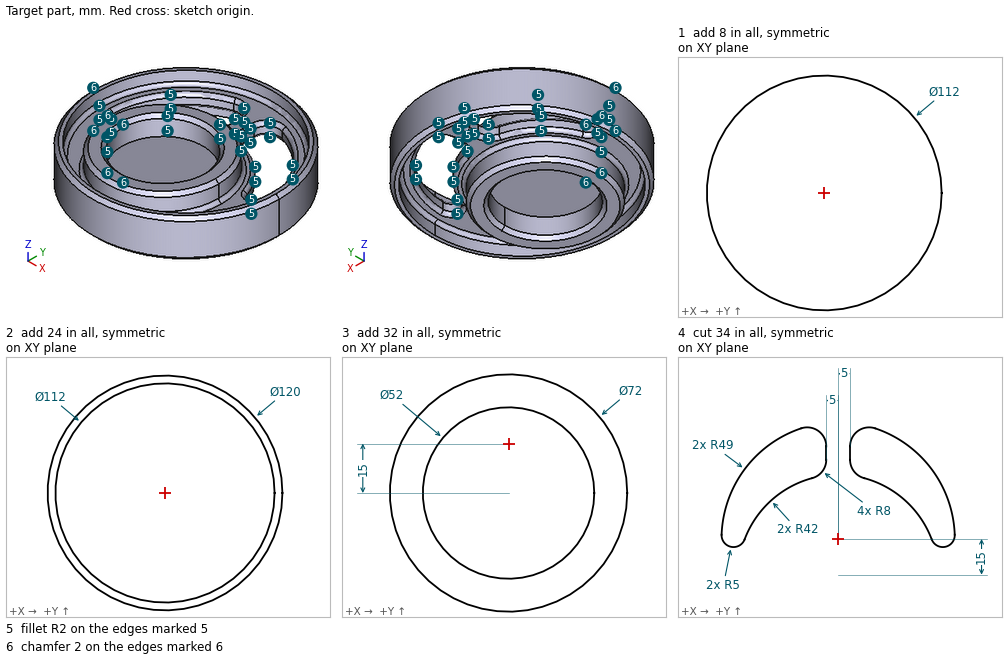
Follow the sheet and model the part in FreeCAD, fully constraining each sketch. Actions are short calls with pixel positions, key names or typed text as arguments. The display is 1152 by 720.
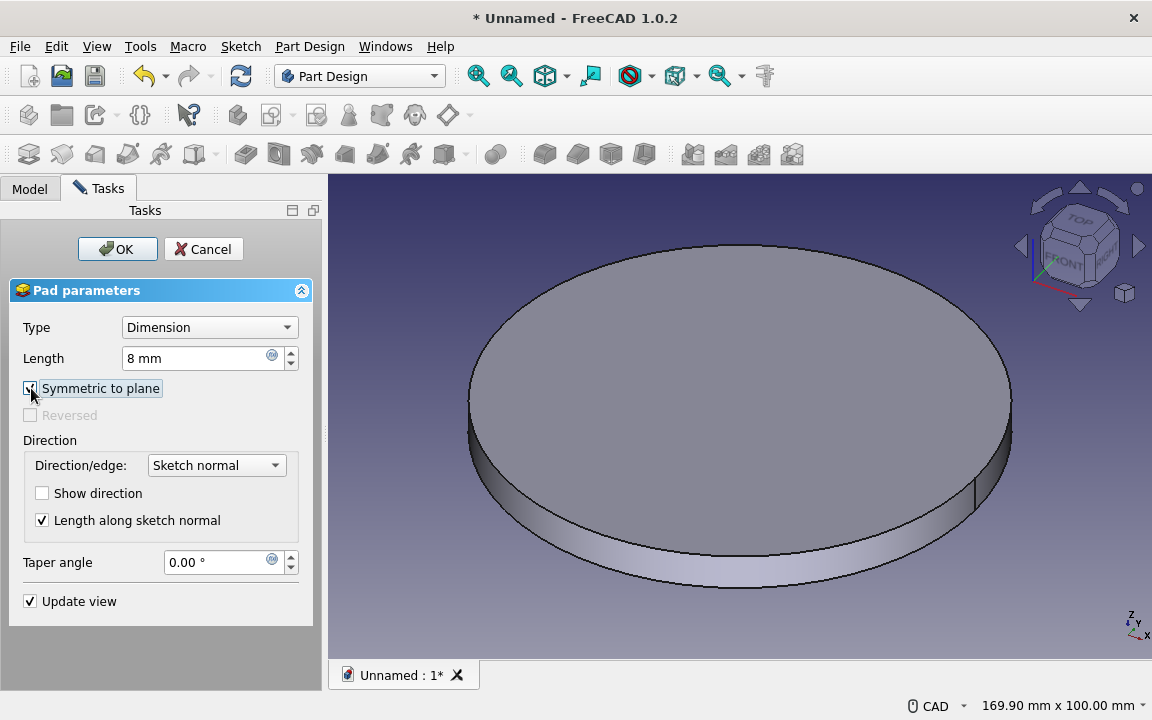
click(118, 249)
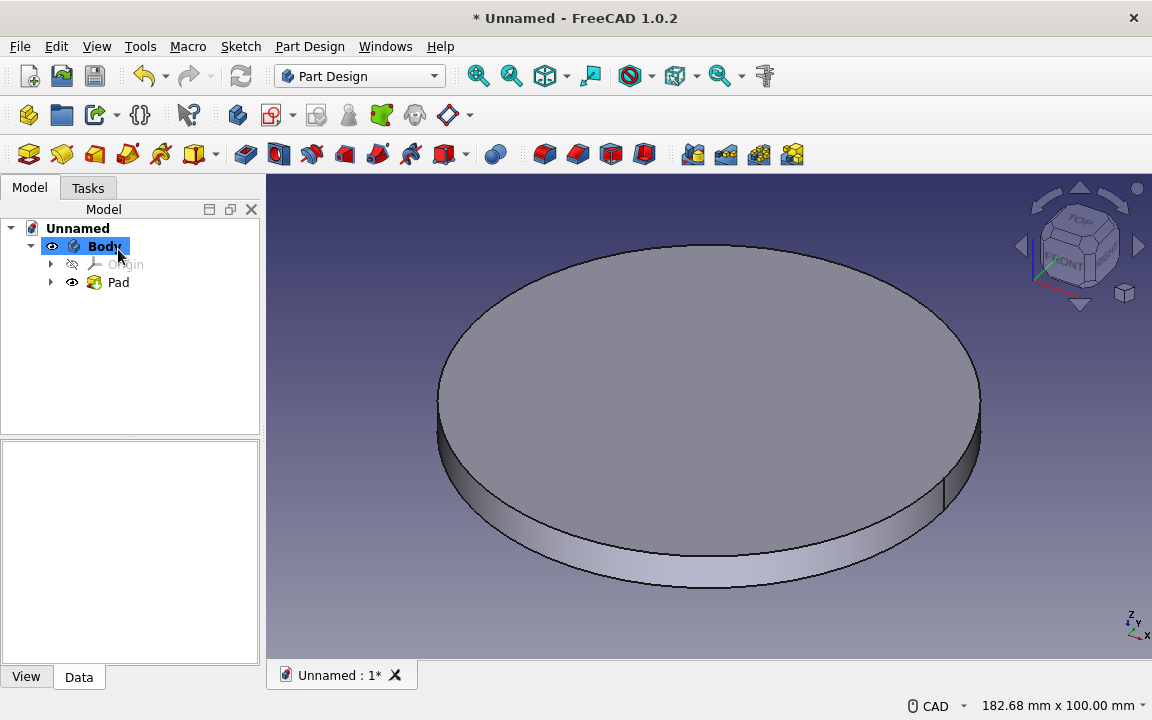
click(270, 116)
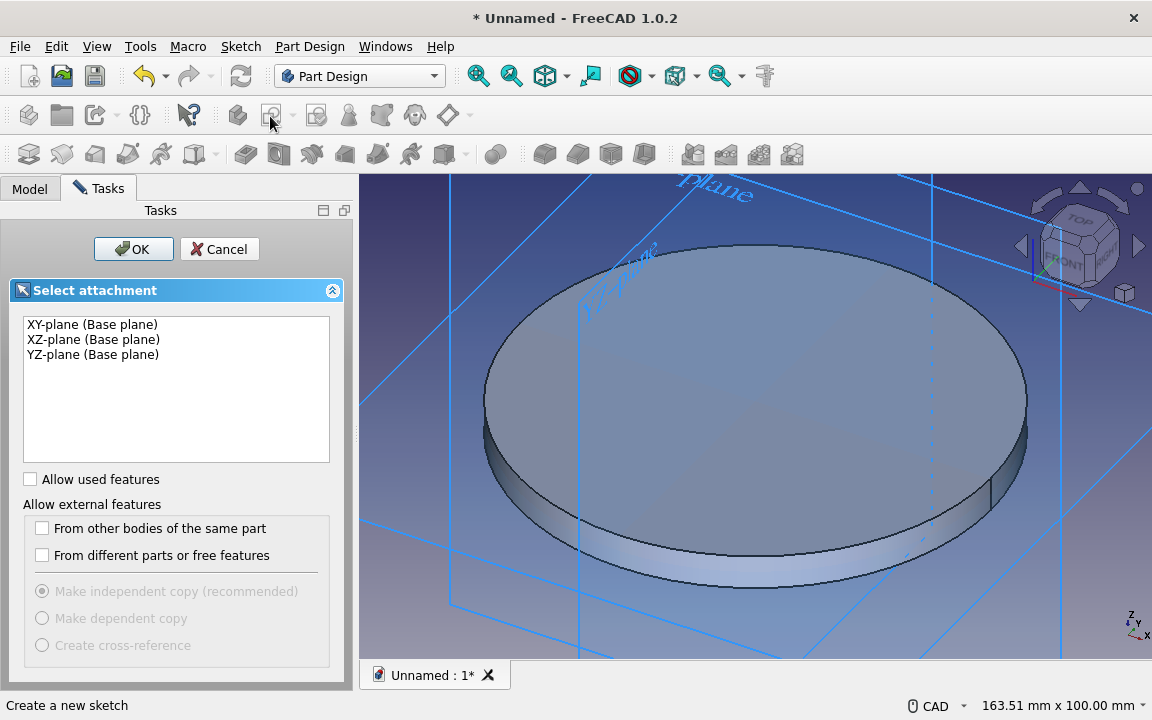
click(84, 324)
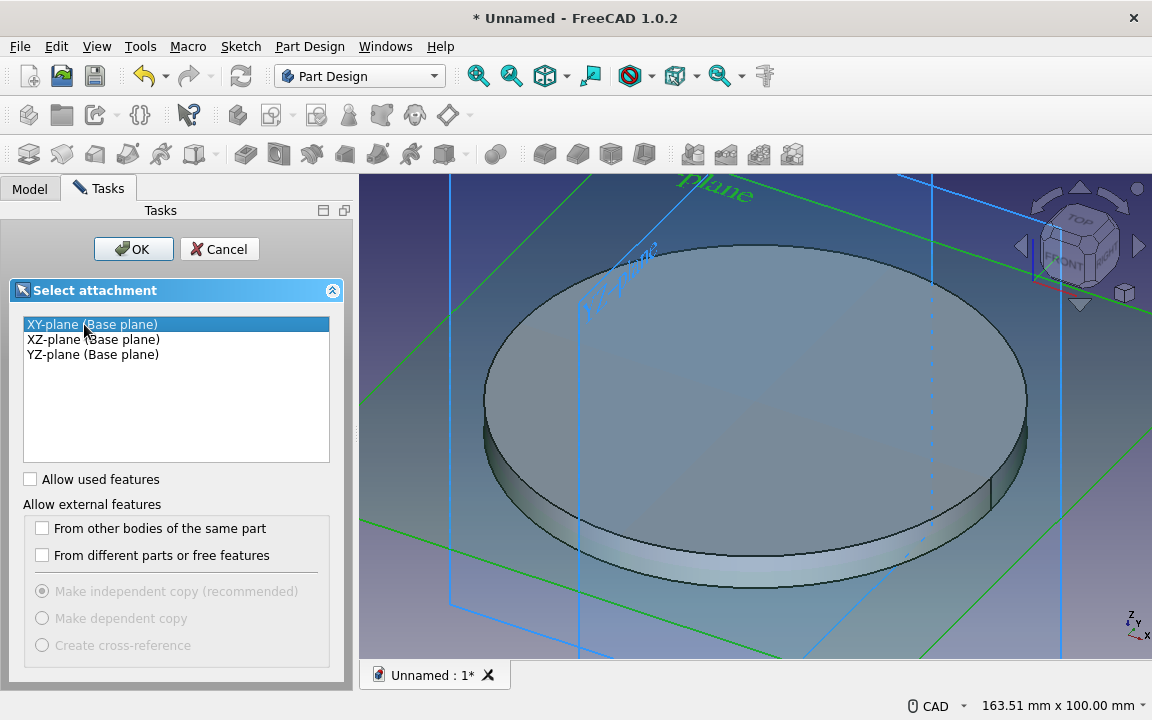
click(134, 249)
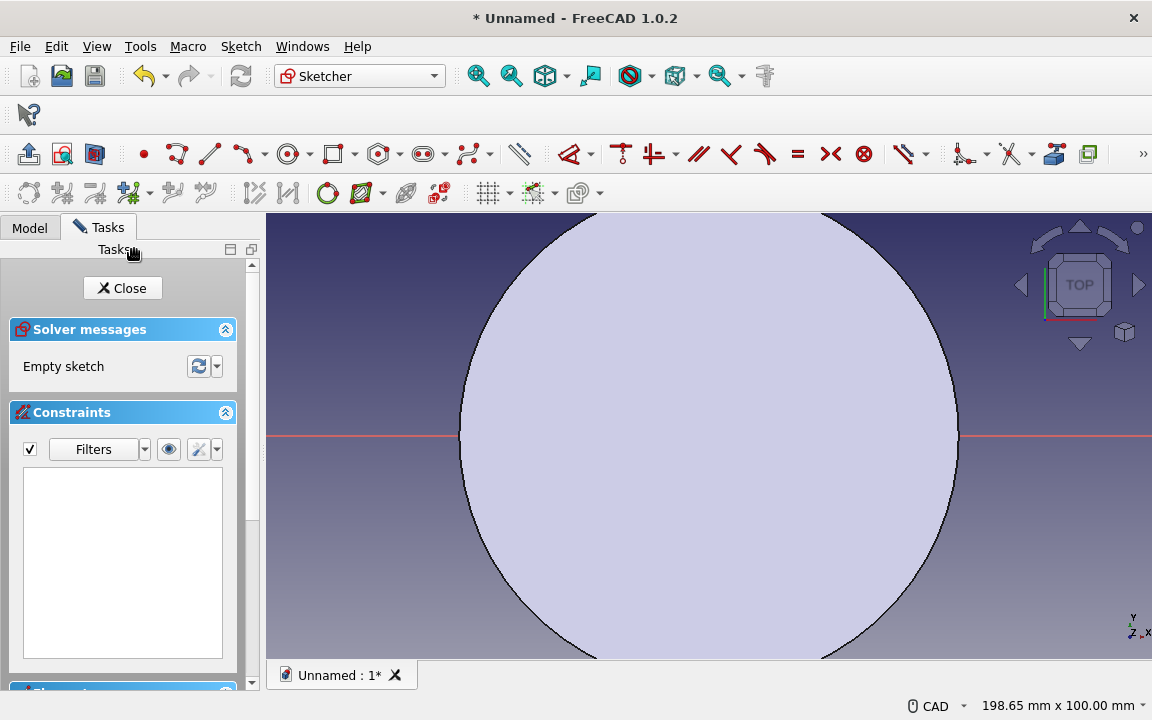
key(q)
key(s)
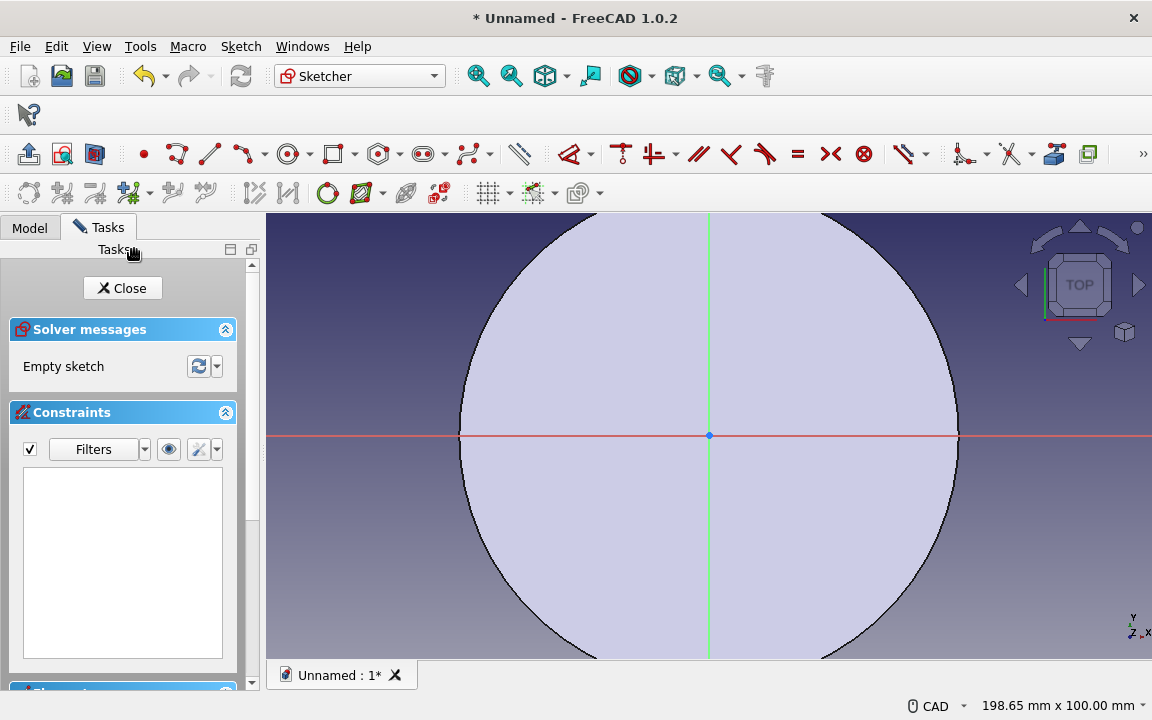
scroll(557, 436, down, 3)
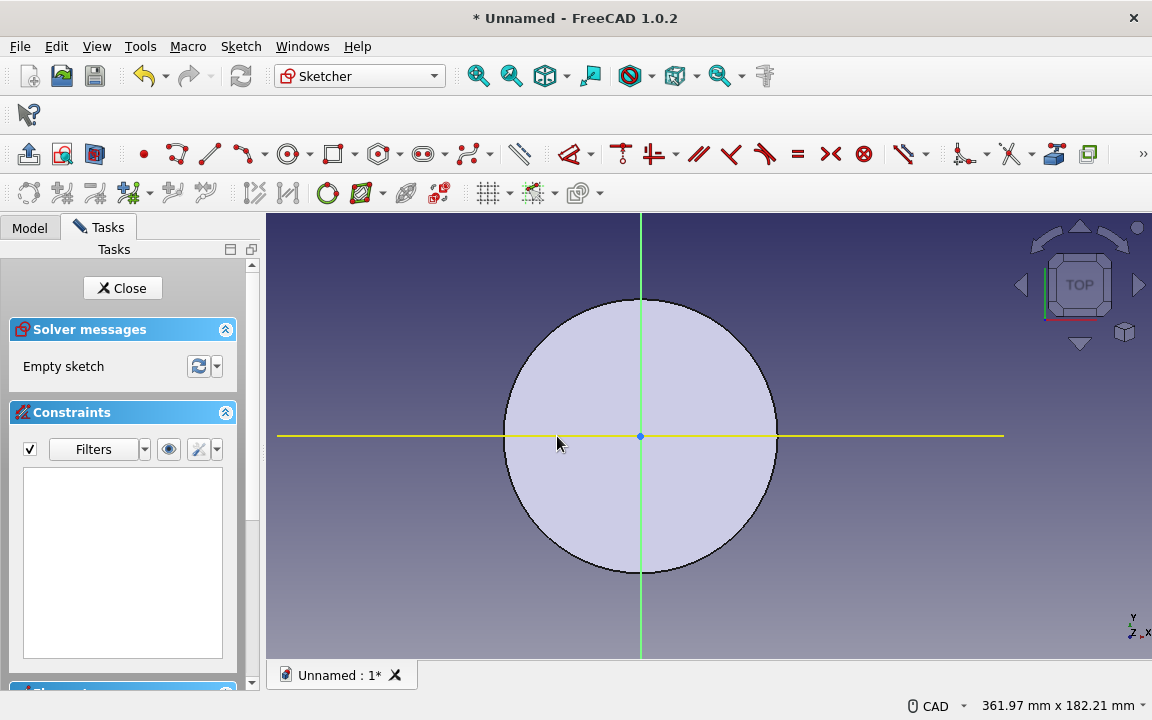
key(g)
key(c)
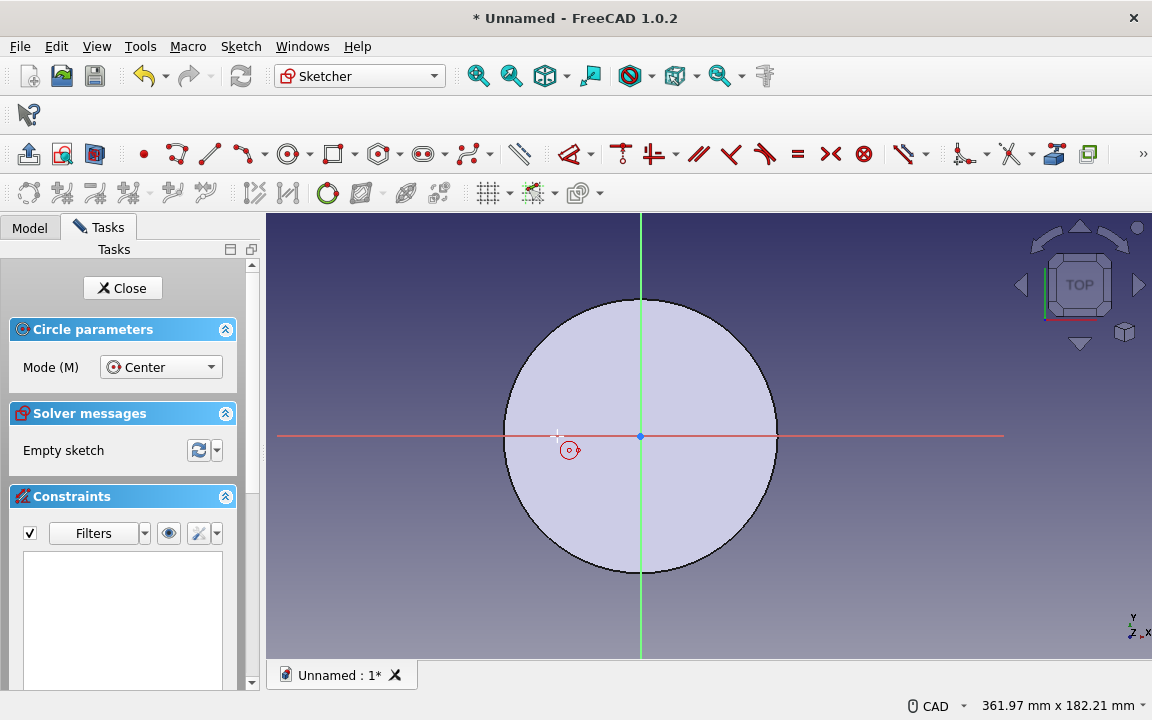
click(641, 436)
move(744, 332)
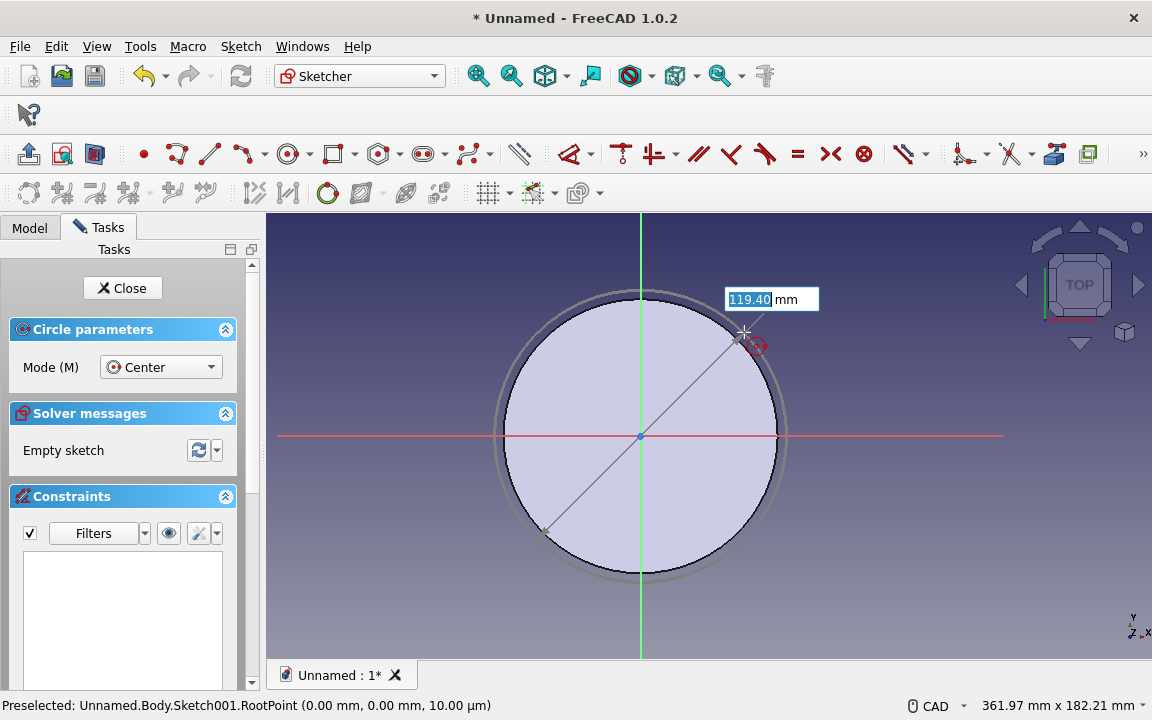
text(120)
key(Return)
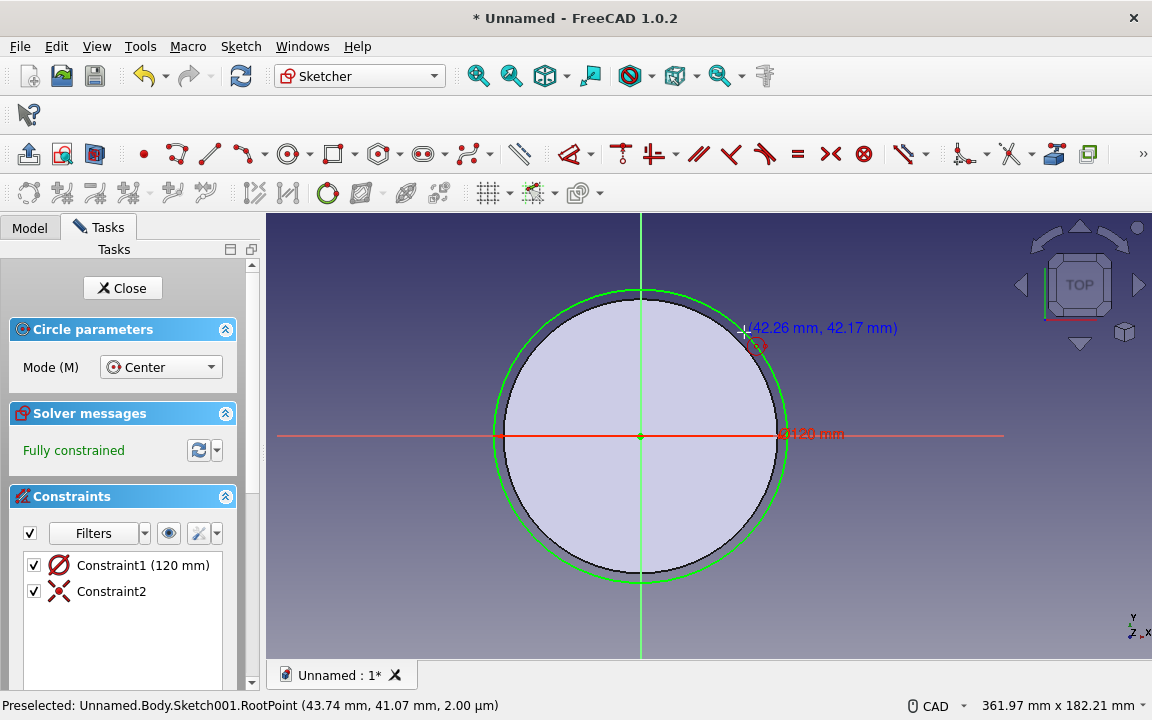
click(641, 436)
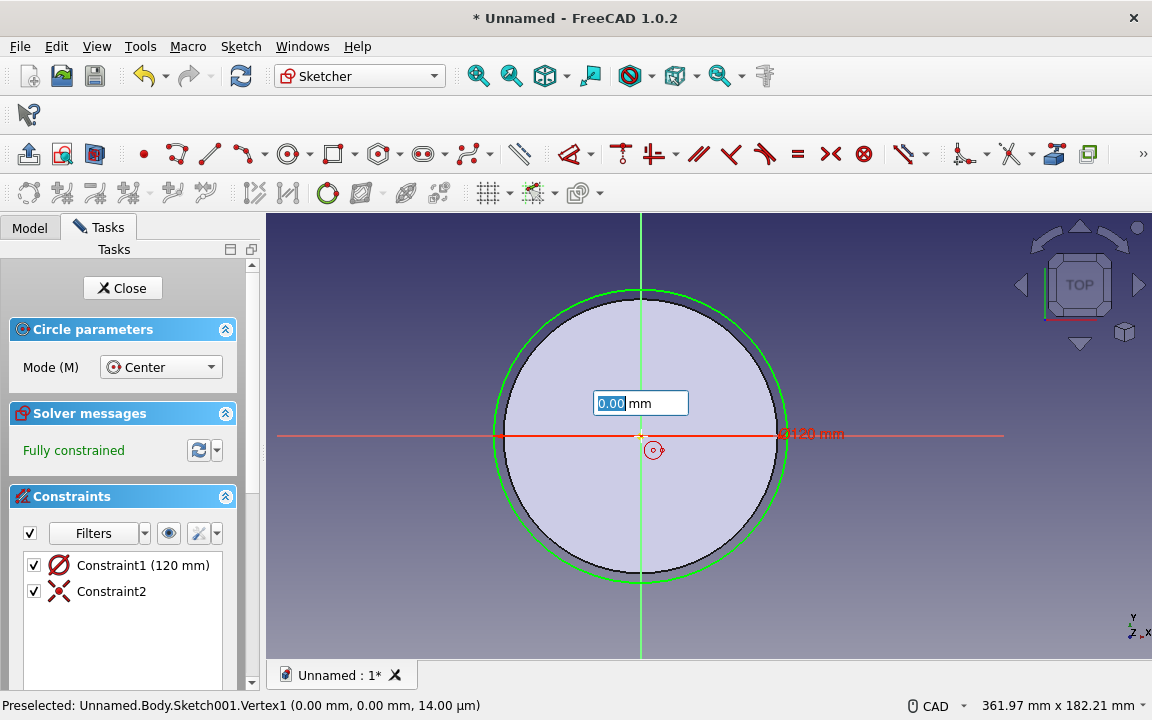
scroll(737, 339, up, 3)
move(737, 339)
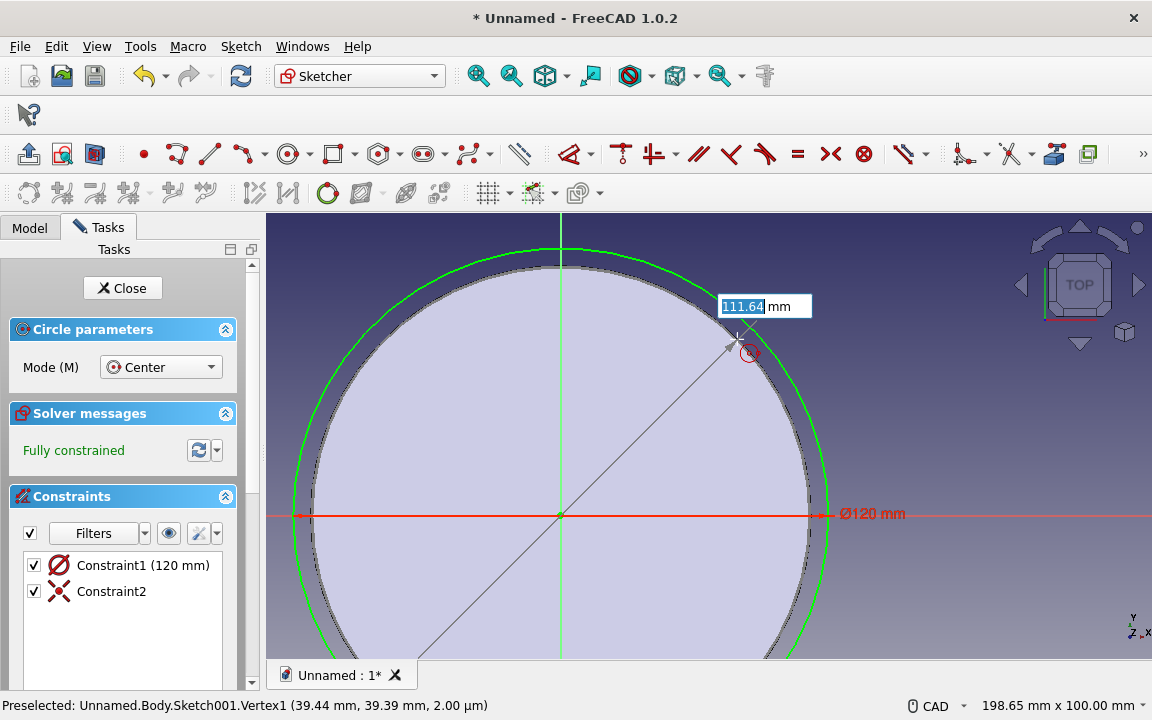
text(112)
key(Return)
key(Escape)